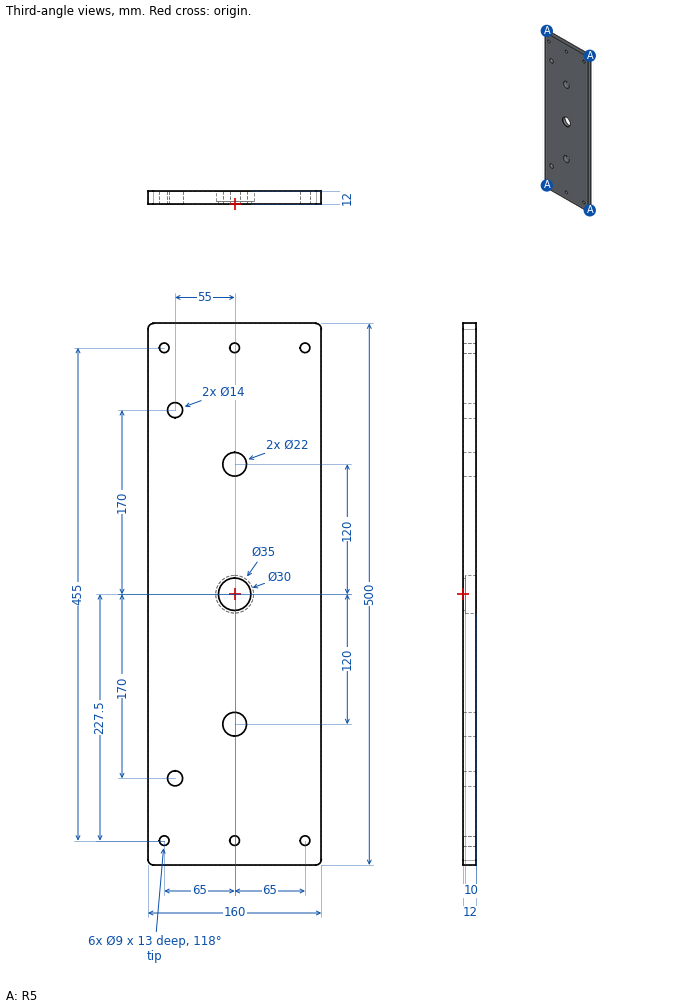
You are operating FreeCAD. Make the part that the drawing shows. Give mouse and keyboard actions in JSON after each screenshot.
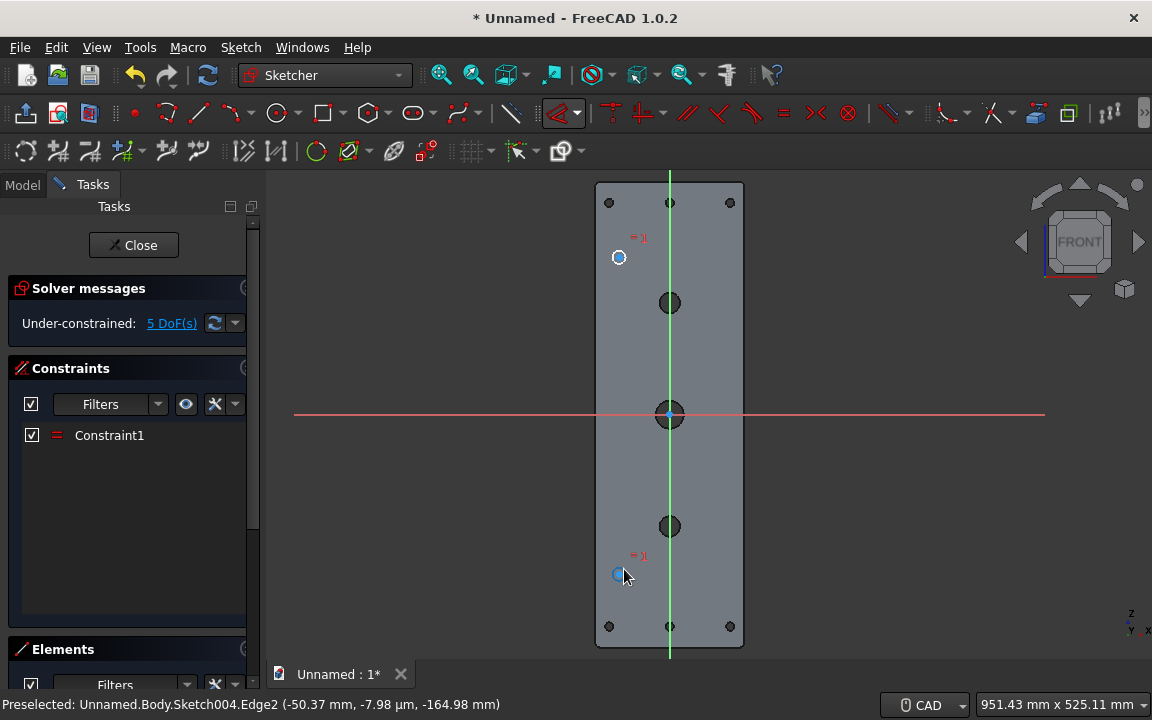
{"action": "scroll", "coordinate": [624, 253], "scroll_direction": "up", "scroll_amount": 6}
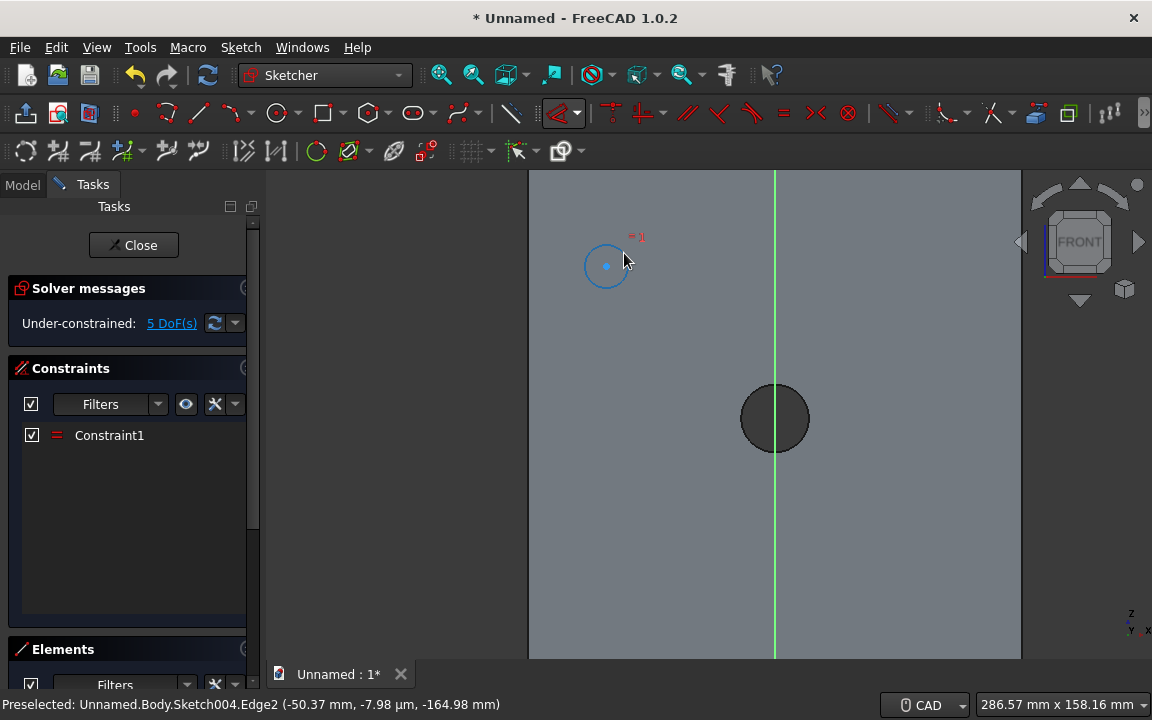
{"action": "left_click", "coordinate": [622, 251]}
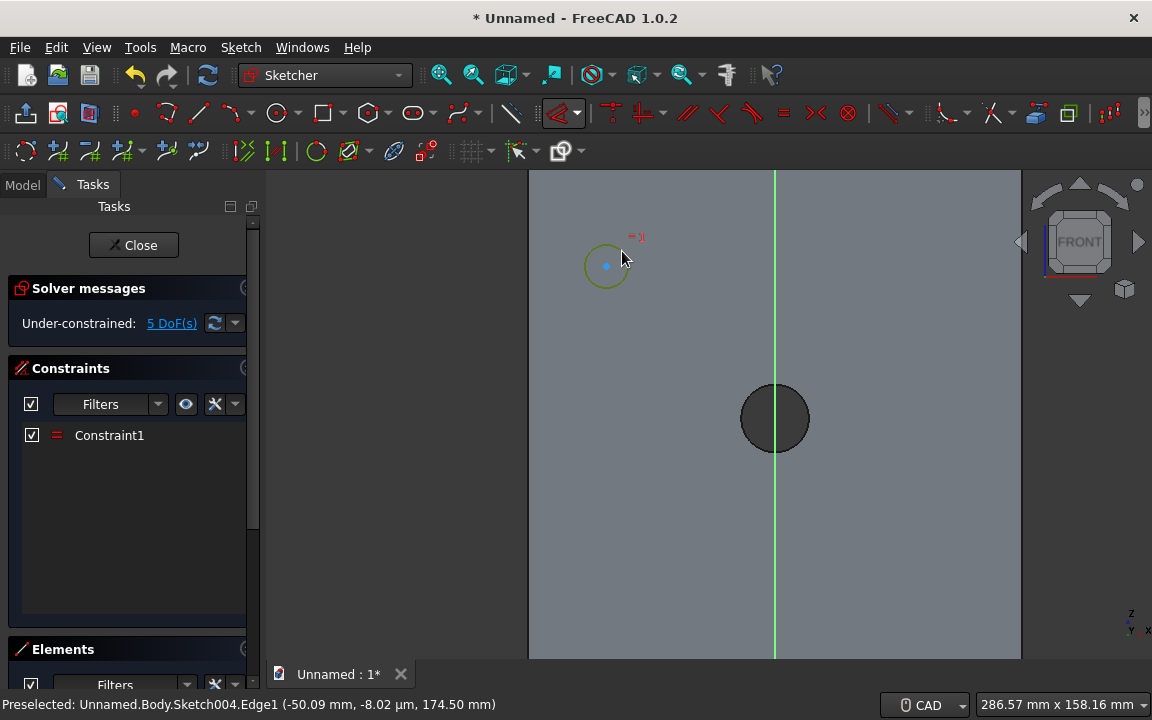
{"action": "key", "text": "k o"}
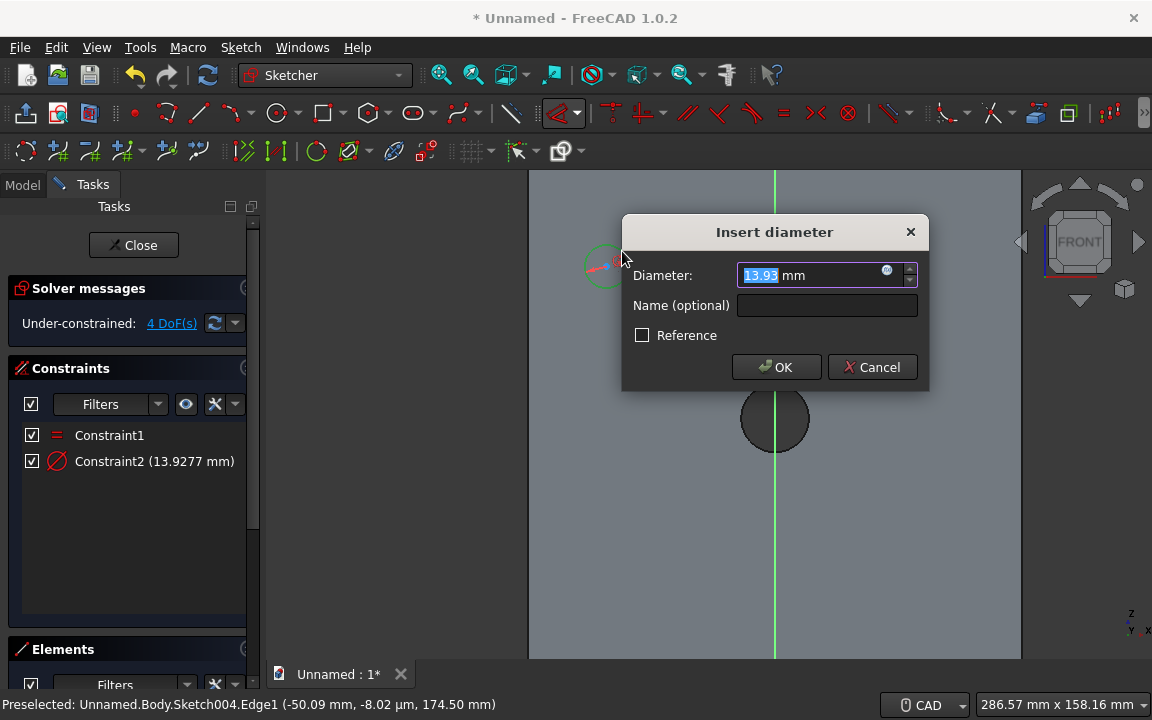
{"action": "type", "text": "14"}
{"action": "key", "text": "Return"}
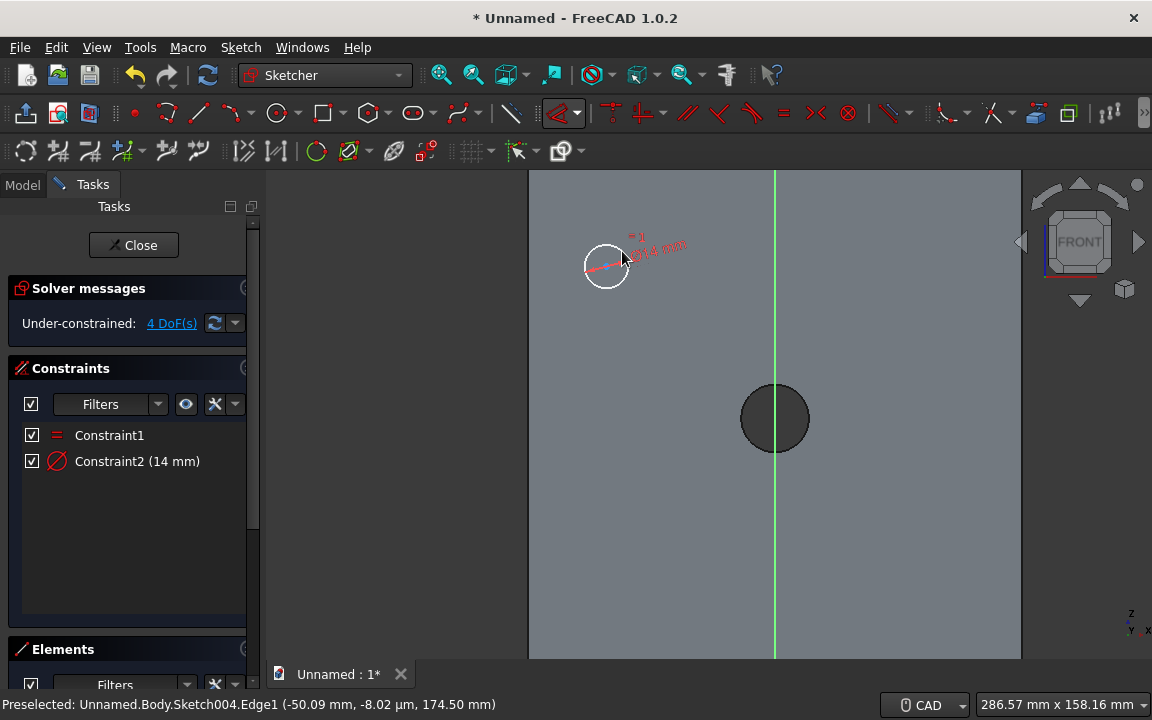
{"action": "left_click", "coordinate": [606, 267]}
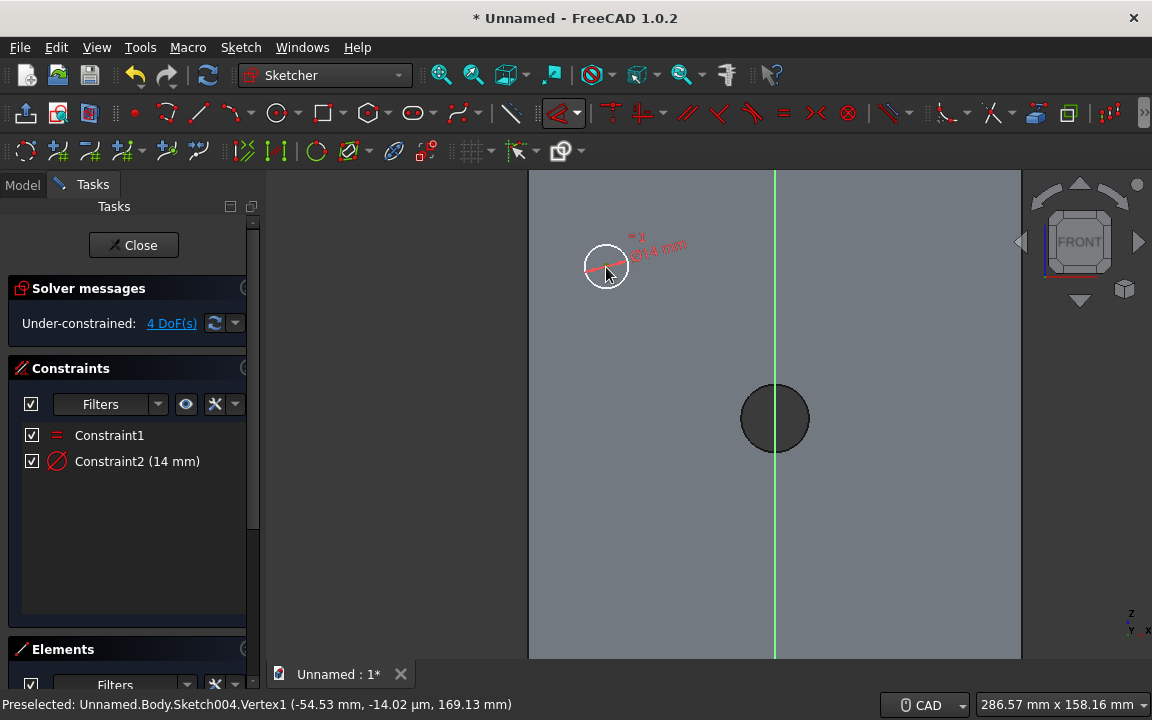
{"action": "key", "text": "l"}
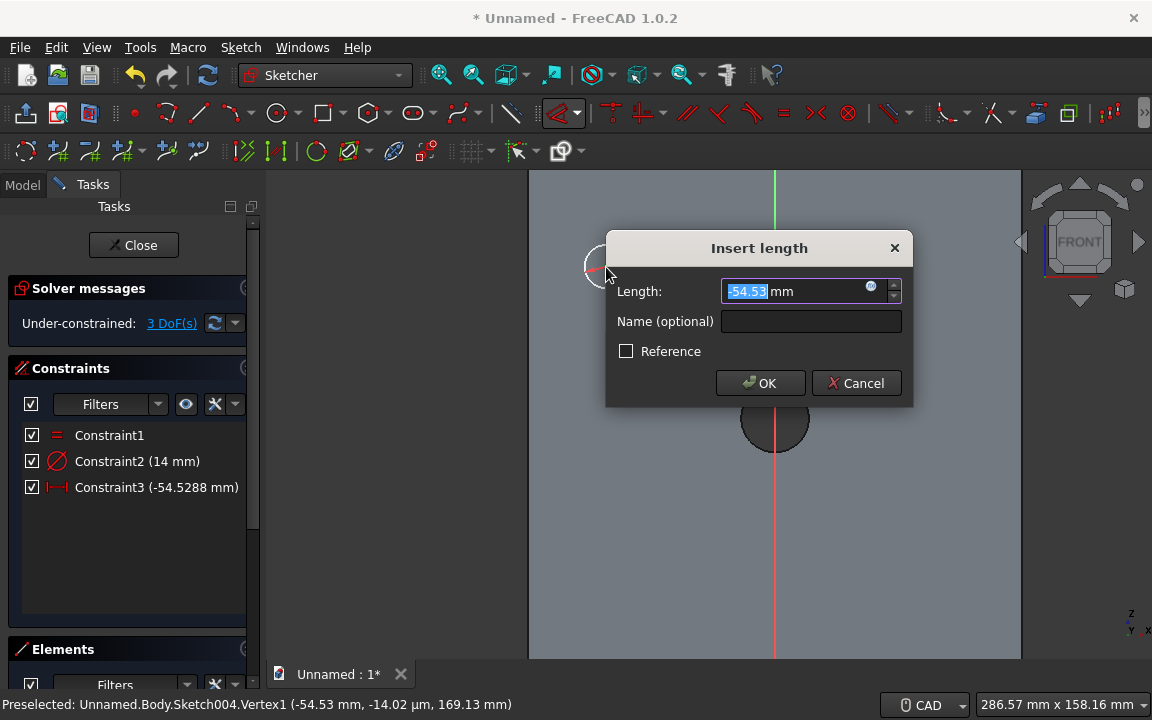
{"action": "type", "text": "-55"}
{"action": "key", "text": "Return"}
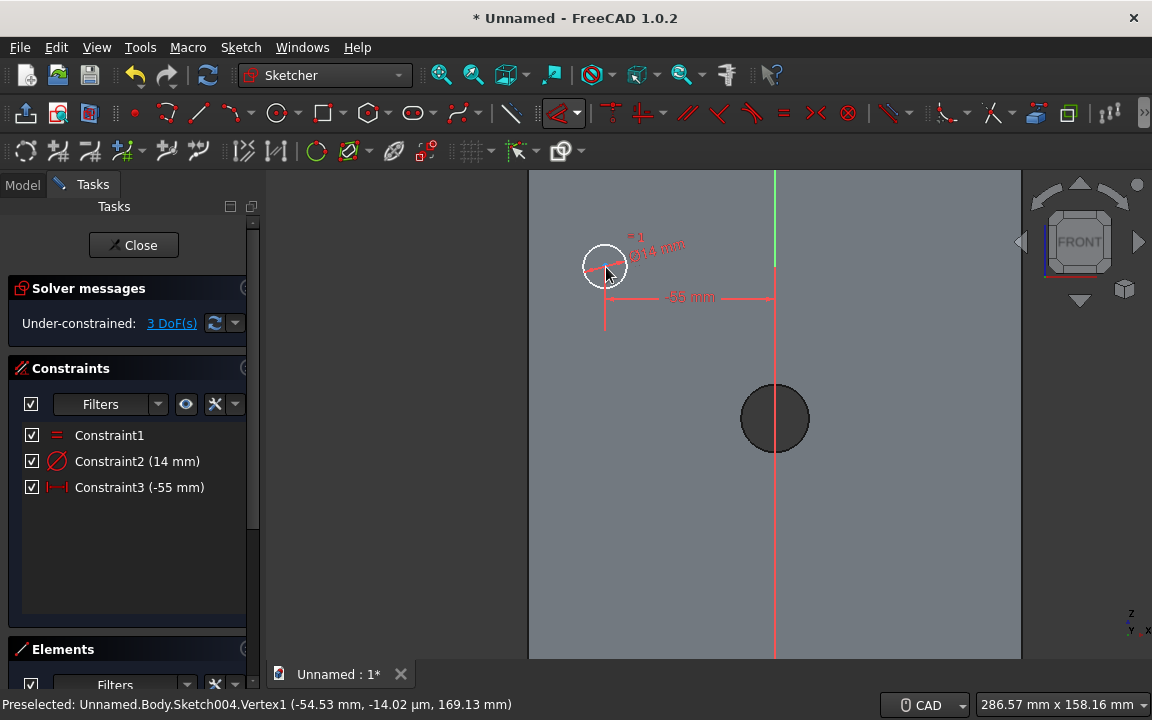
{"action": "scroll", "coordinate": [624, 253], "scroll_direction": "down", "scroll_amount": 6}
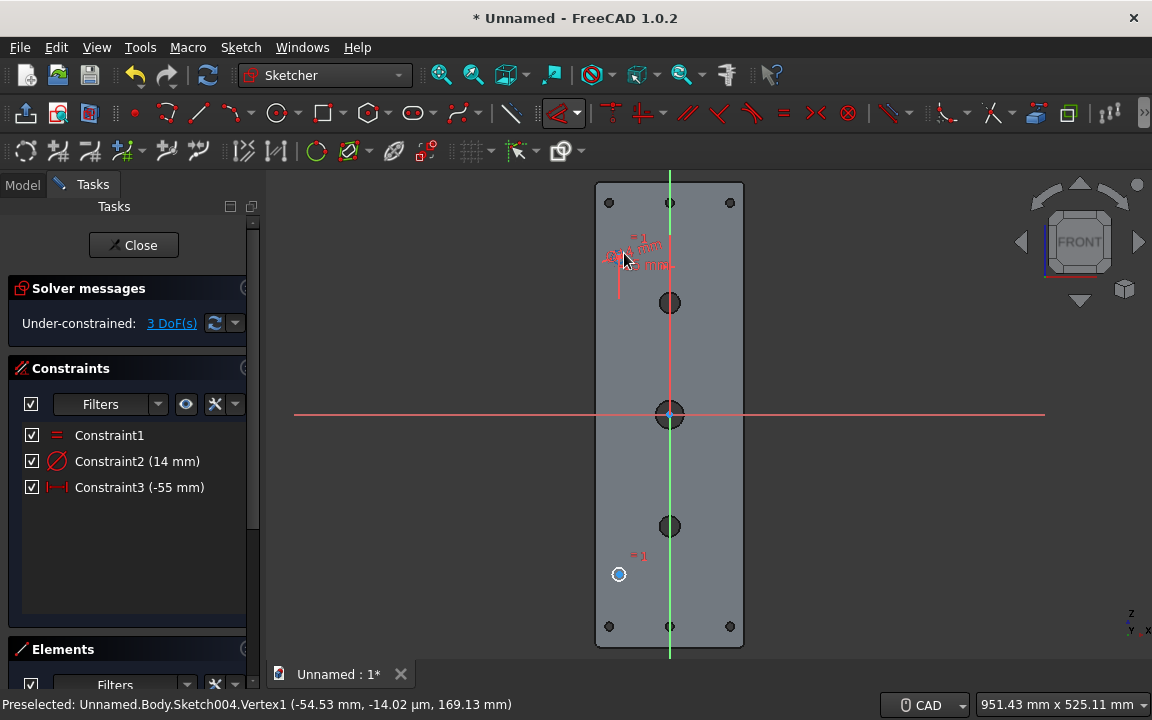
{"action": "left_click", "coordinate": [619, 574]}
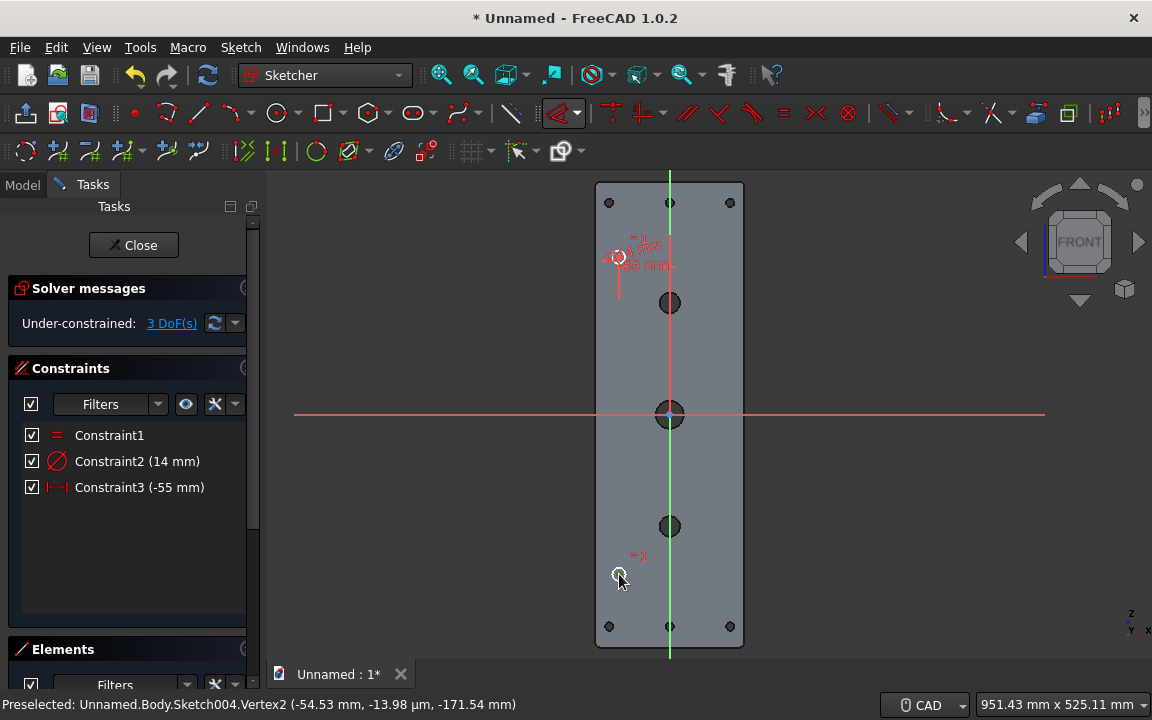
{"action": "left_click", "coordinate": [580, 114]}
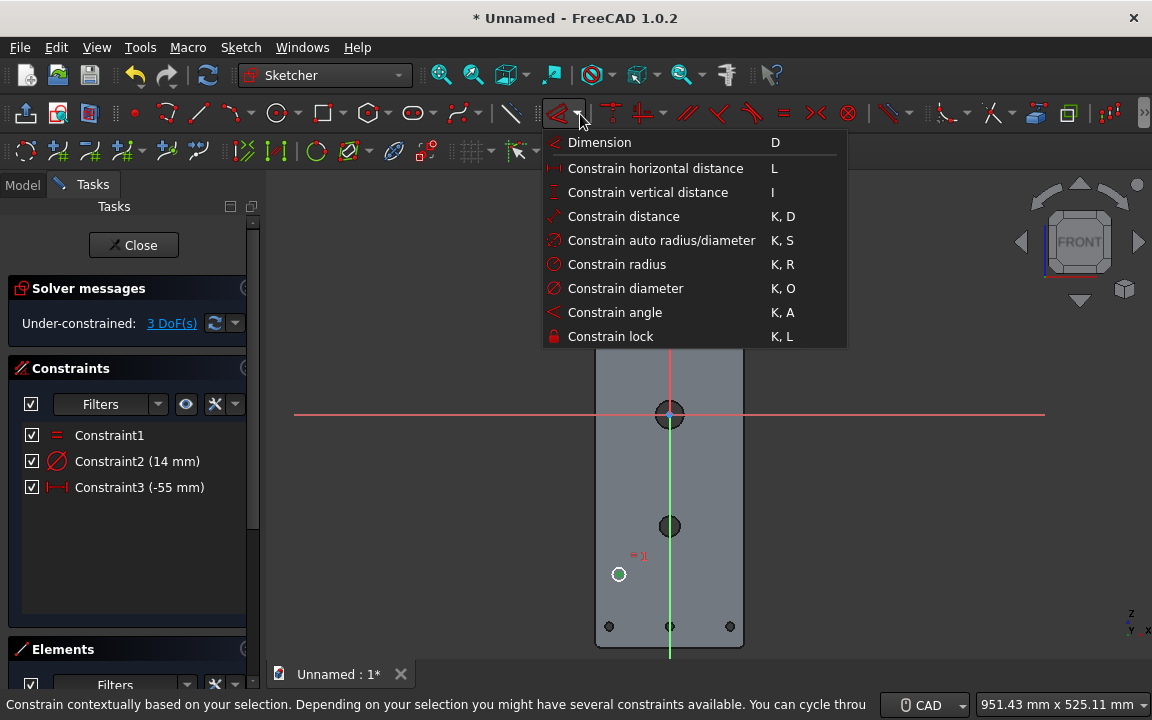
{"action": "left_click", "coordinate": [695, 168]}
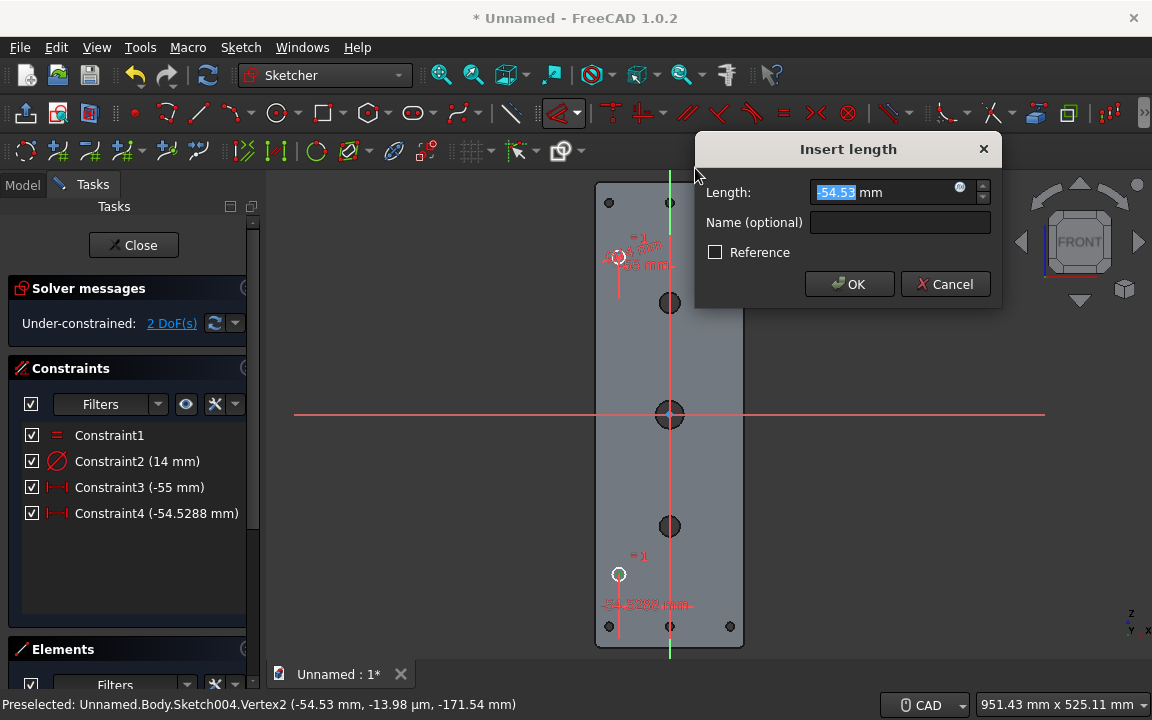
{"action": "type", "text": "-55"}
{"action": "key", "text": "Return"}